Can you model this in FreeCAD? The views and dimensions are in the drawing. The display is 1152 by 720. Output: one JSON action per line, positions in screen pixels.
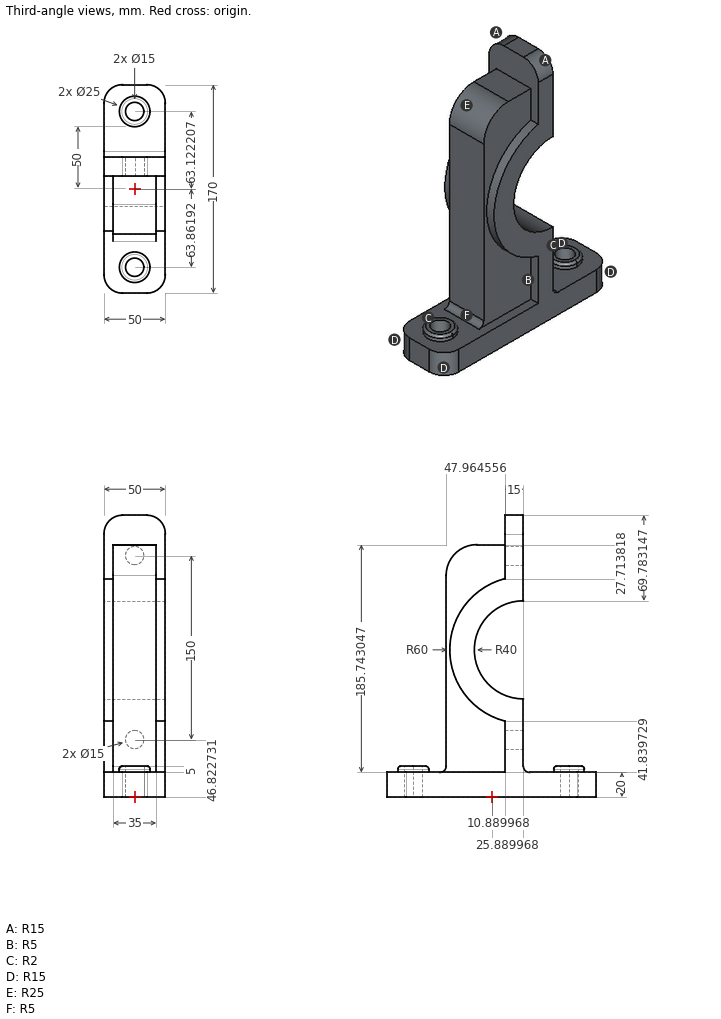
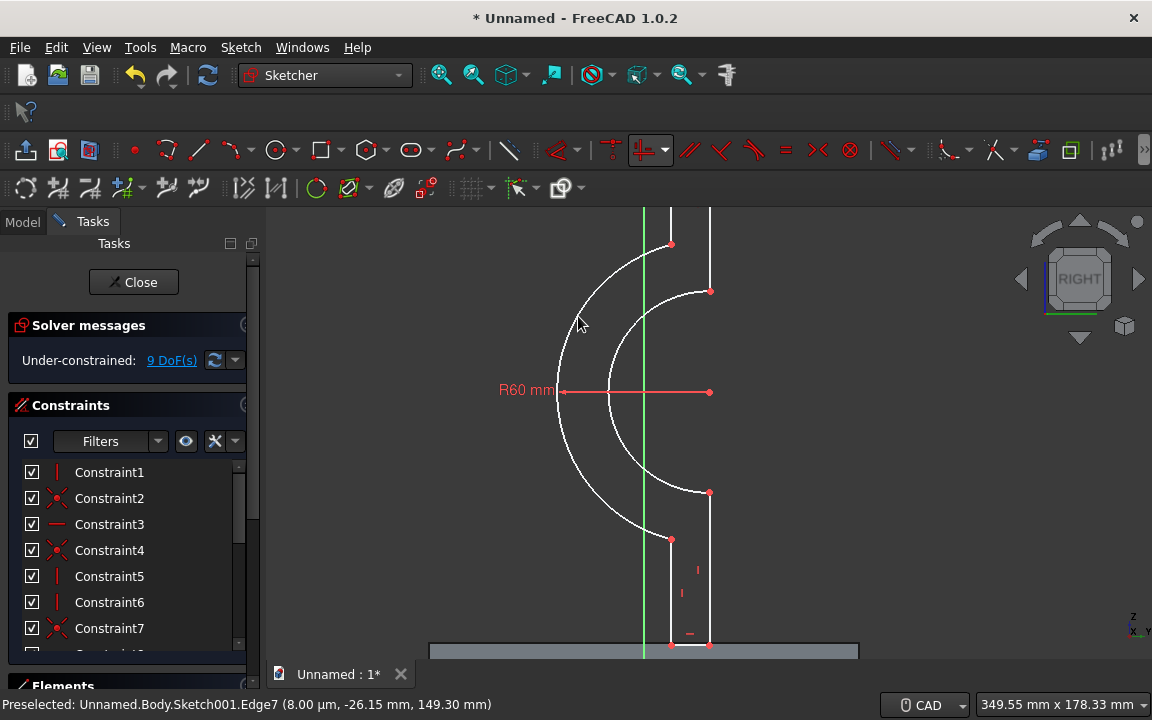
{"action": "left_click", "coordinate": [628, 333]}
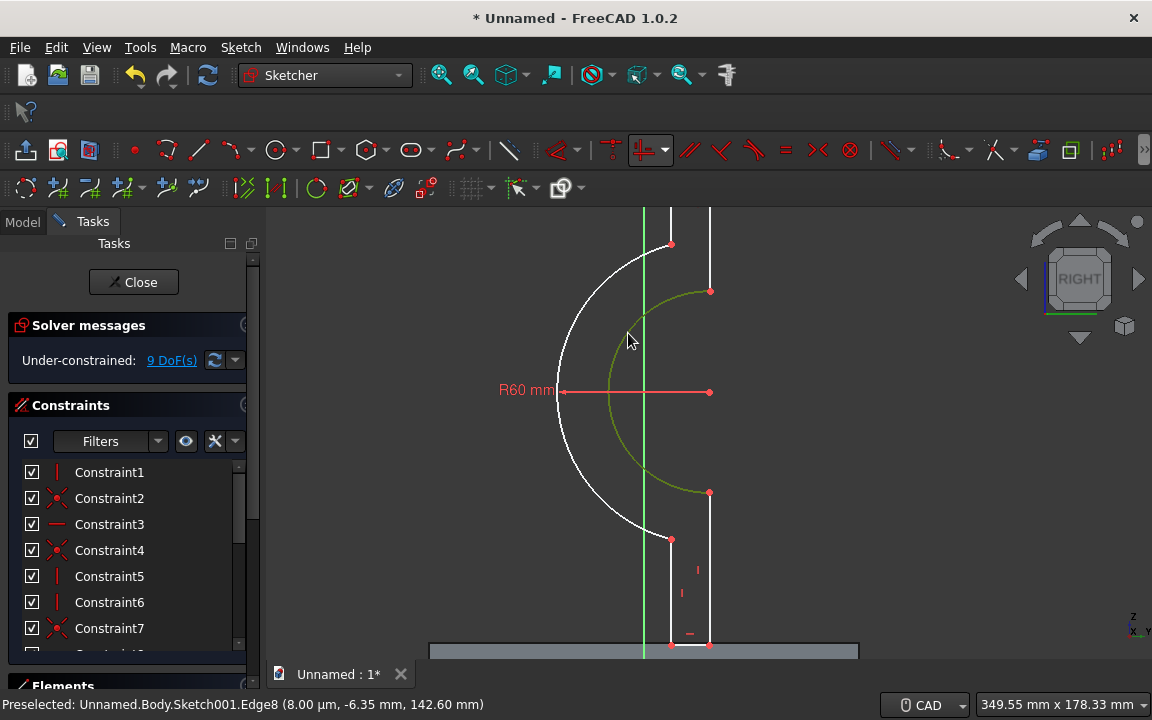
{"action": "key", "text": "k r"}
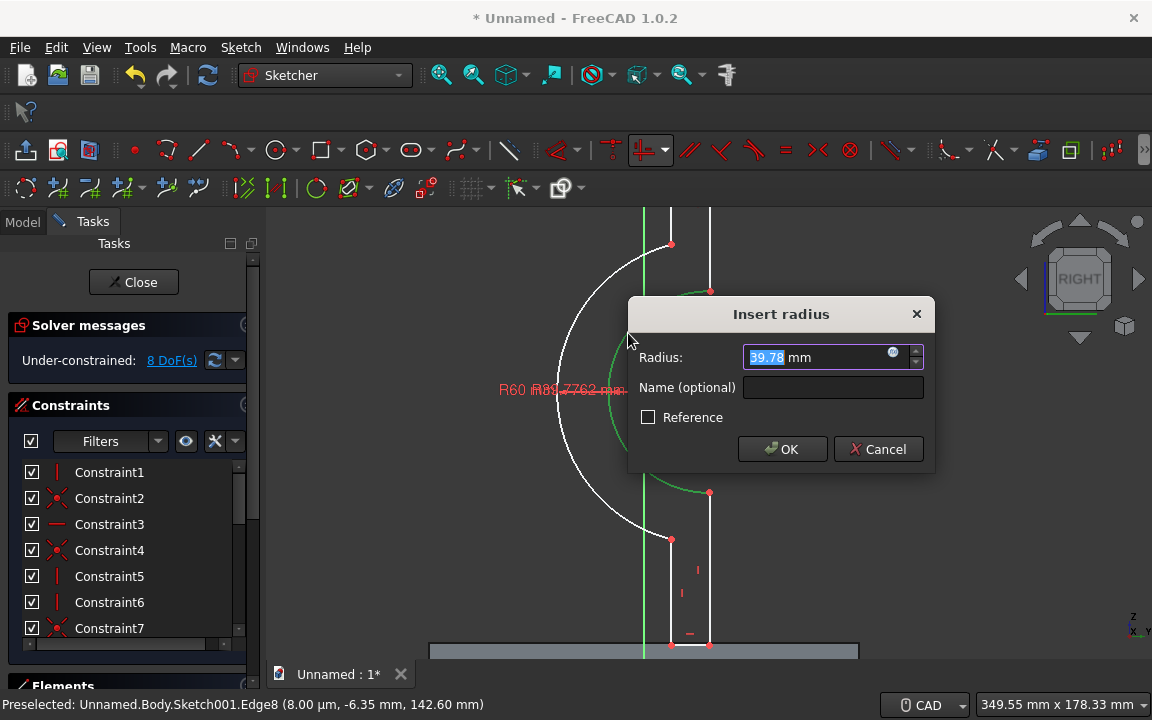
{"action": "type", "text": "40"}
{"action": "key", "text": "Return"}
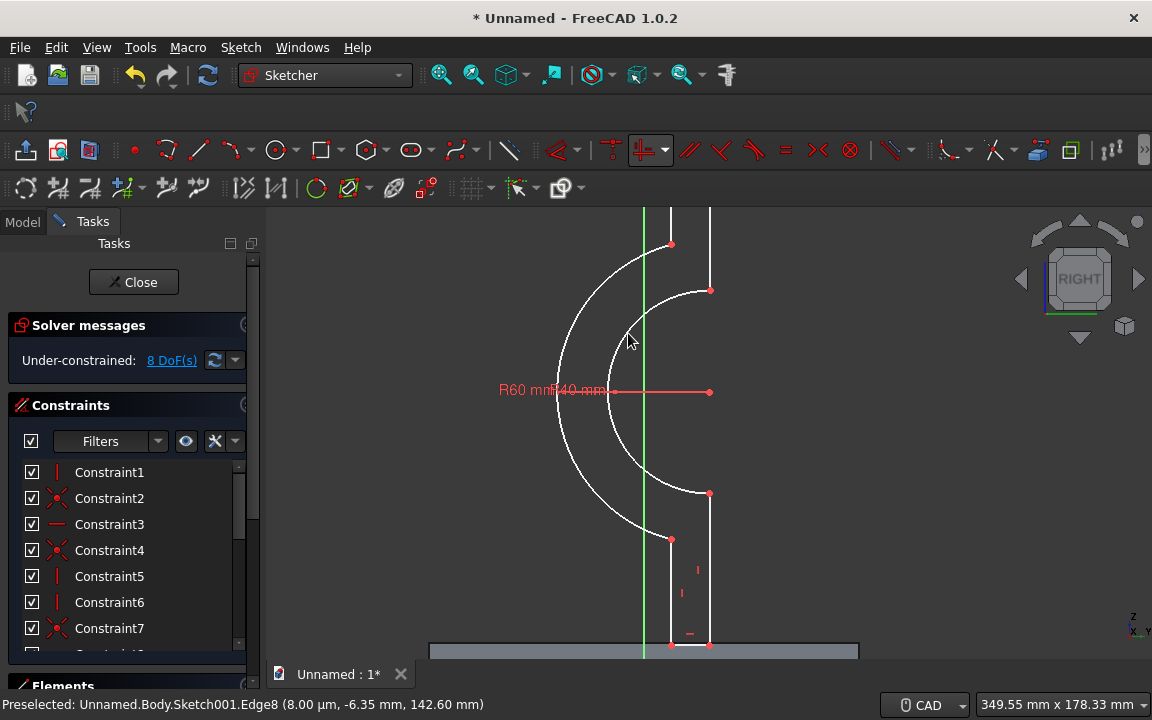
{"action": "scroll", "coordinate": [646, 458], "scroll_direction": "down", "scroll_amount": 4}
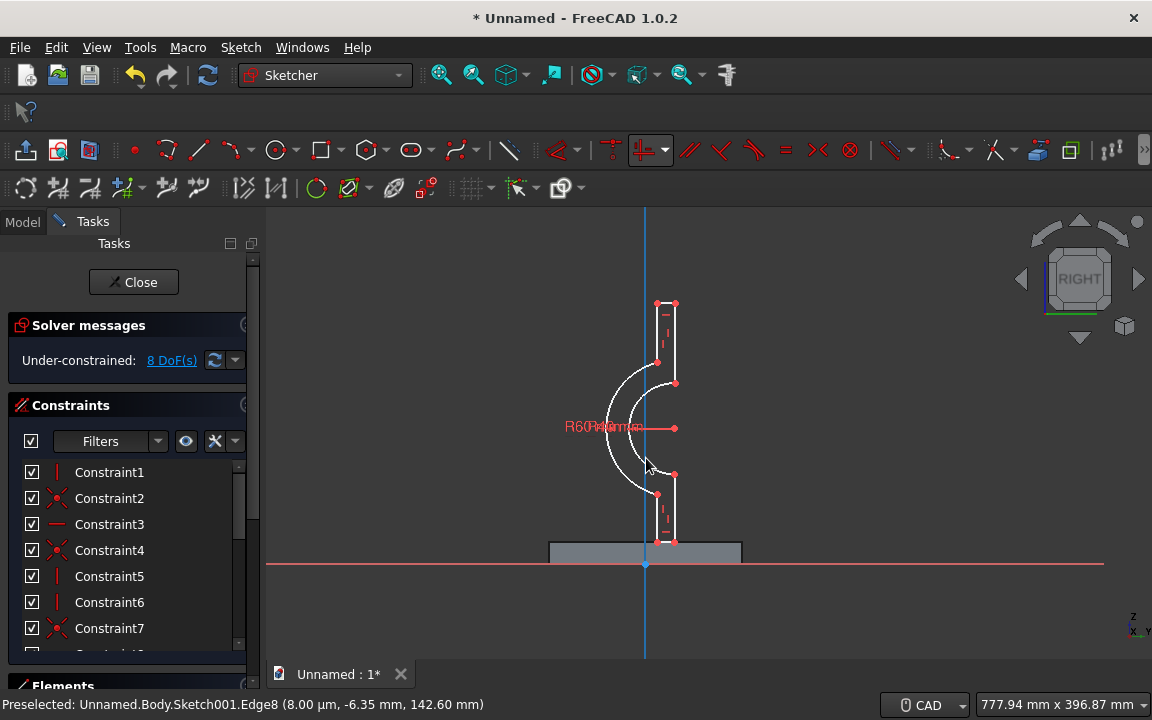
{"action": "scroll", "coordinate": [670, 303], "scroll_direction": "up", "scroll_amount": 5}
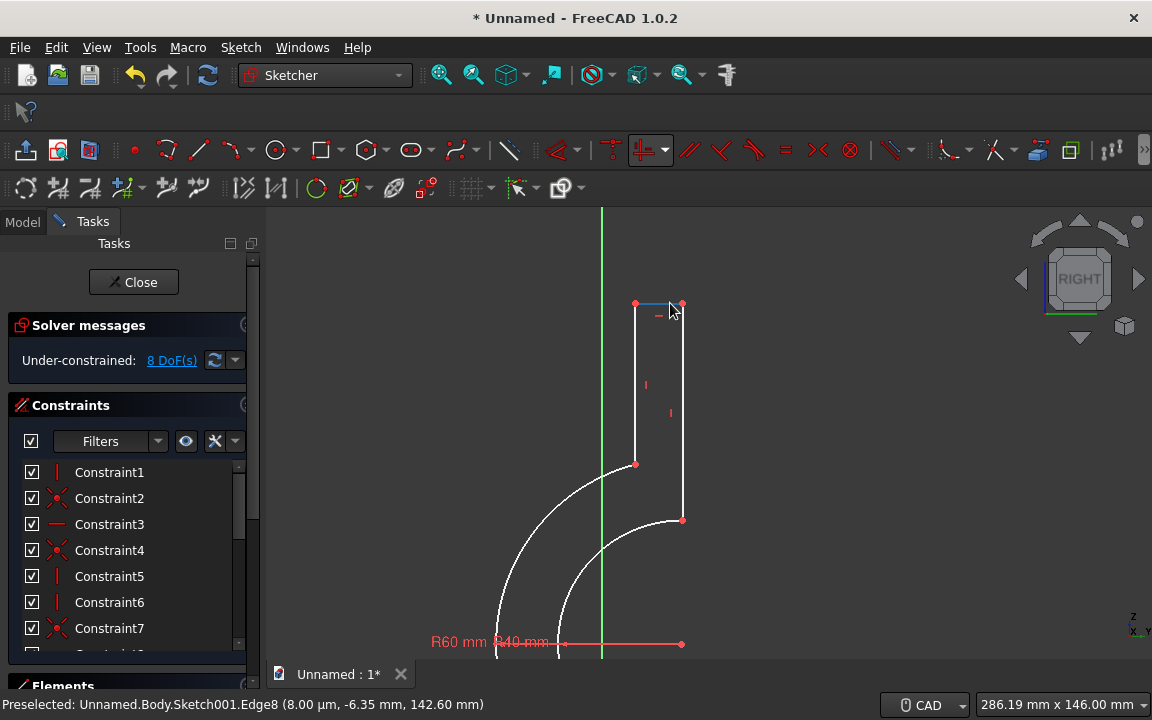
{"action": "left_click", "coordinate": [669, 304]}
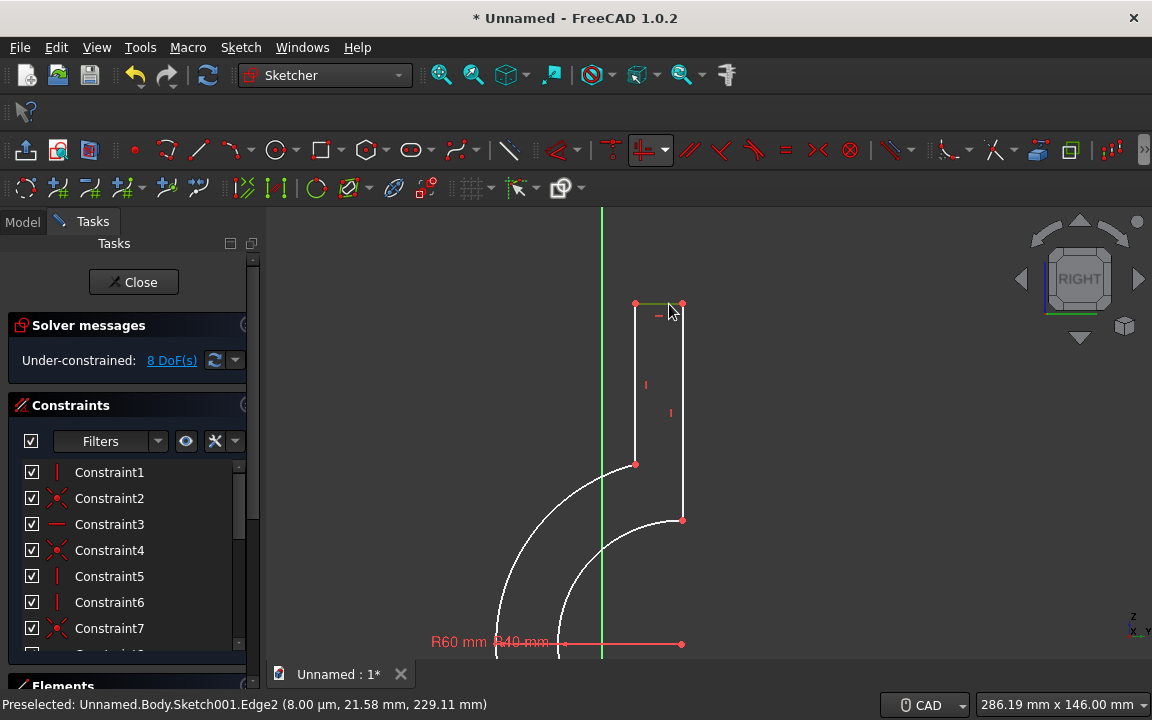
{"action": "key", "text": "l"}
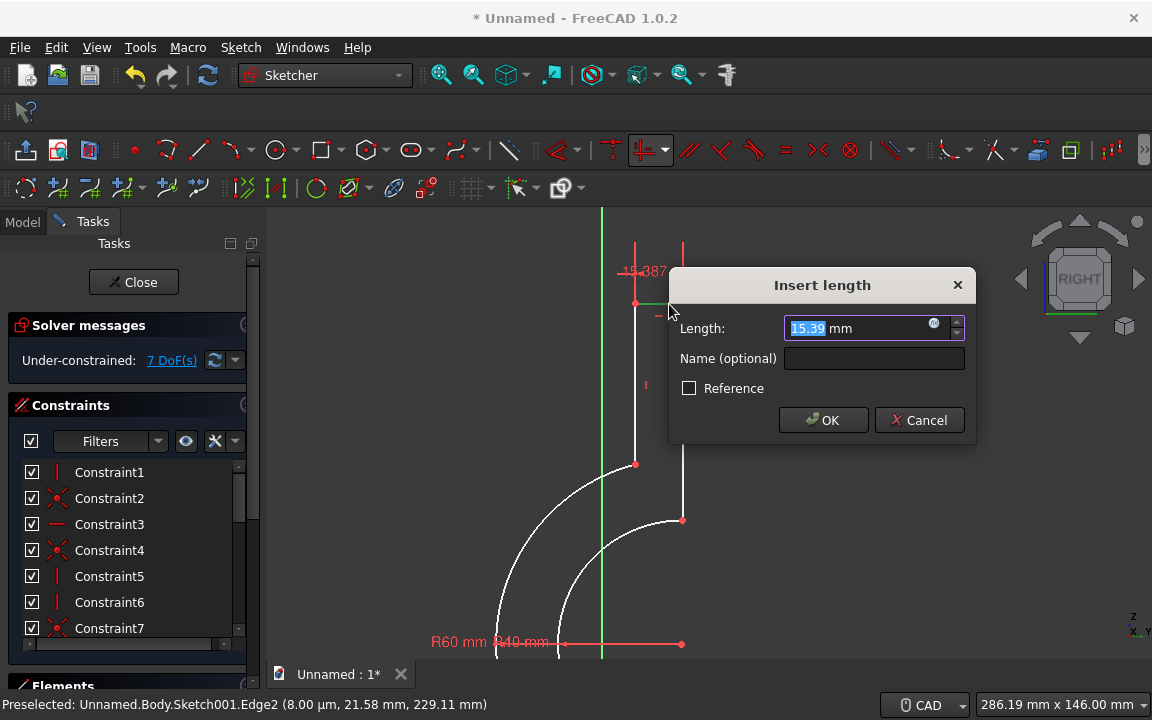
{"action": "type", "text": "15"}
{"action": "key", "text": "Return"}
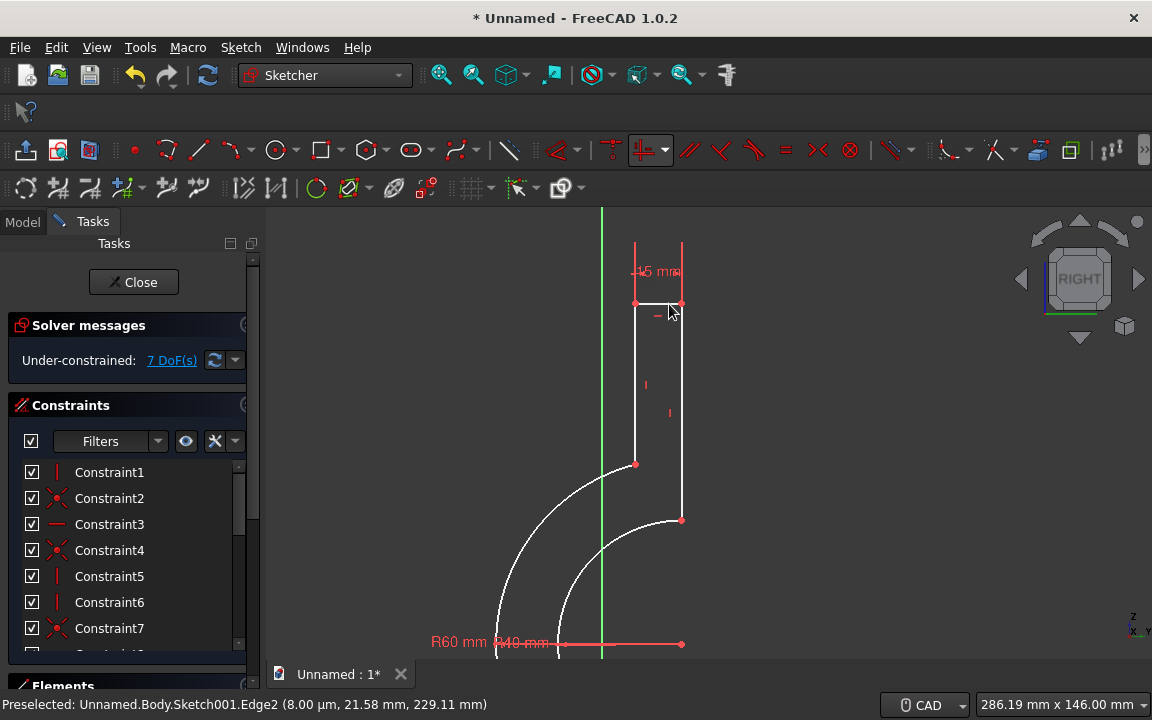
{"action": "scroll", "coordinate": [670, 302], "scroll_direction": "down", "scroll_amount": 5}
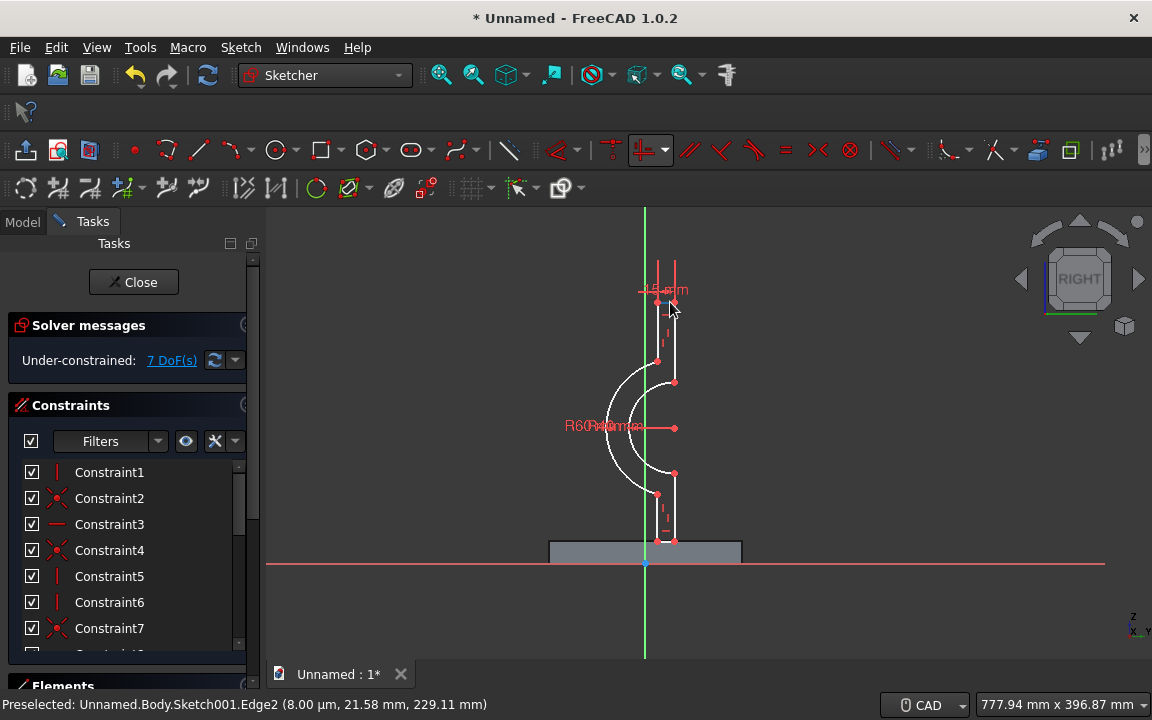
{"action": "scroll", "coordinate": [663, 542], "scroll_direction": "up", "scroll_amount": 5}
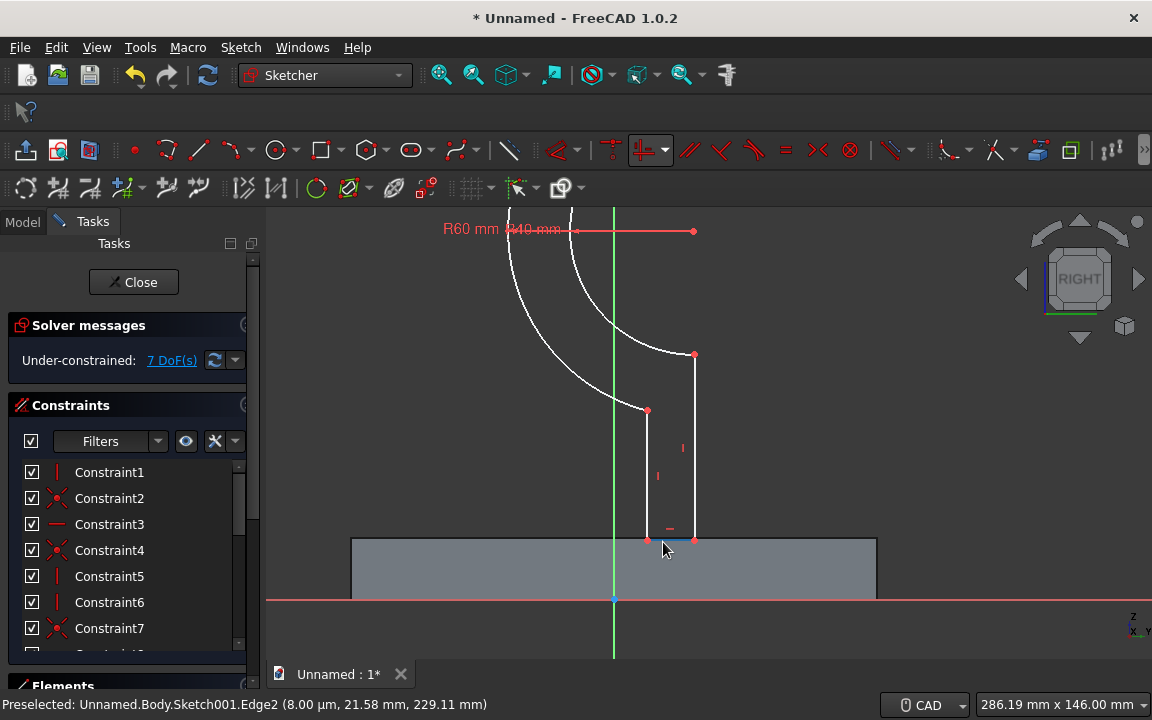
{"action": "left_click", "coordinate": [661, 540]}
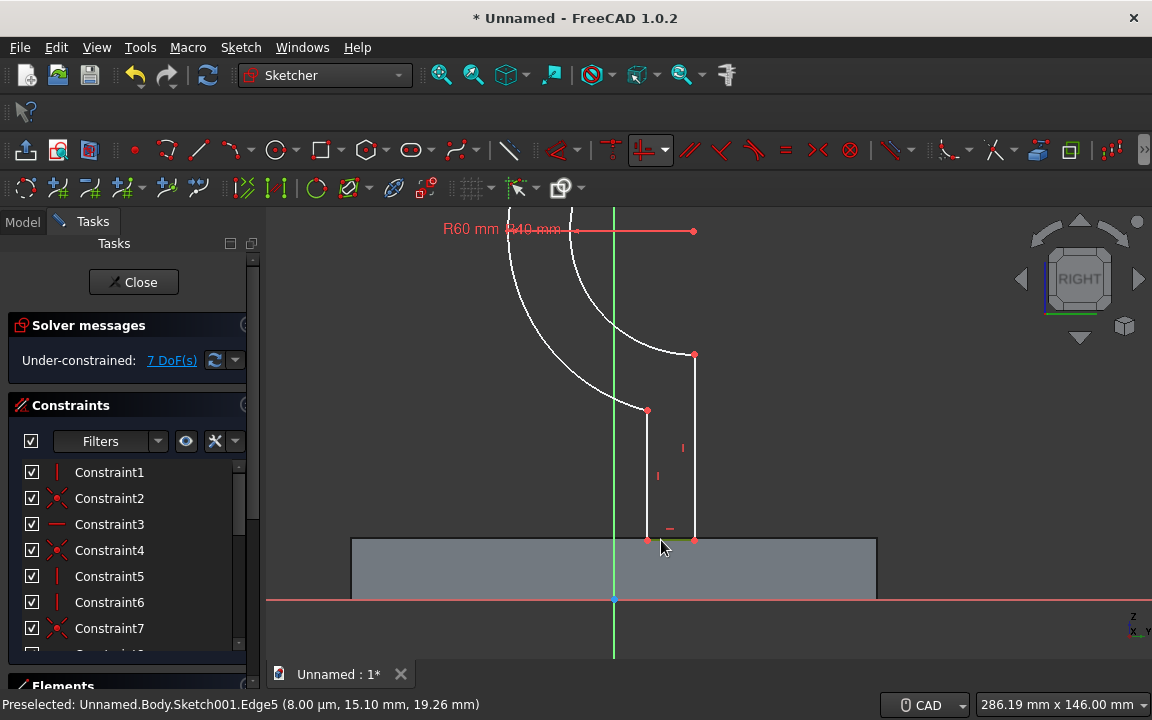
{"action": "key", "text": "l"}